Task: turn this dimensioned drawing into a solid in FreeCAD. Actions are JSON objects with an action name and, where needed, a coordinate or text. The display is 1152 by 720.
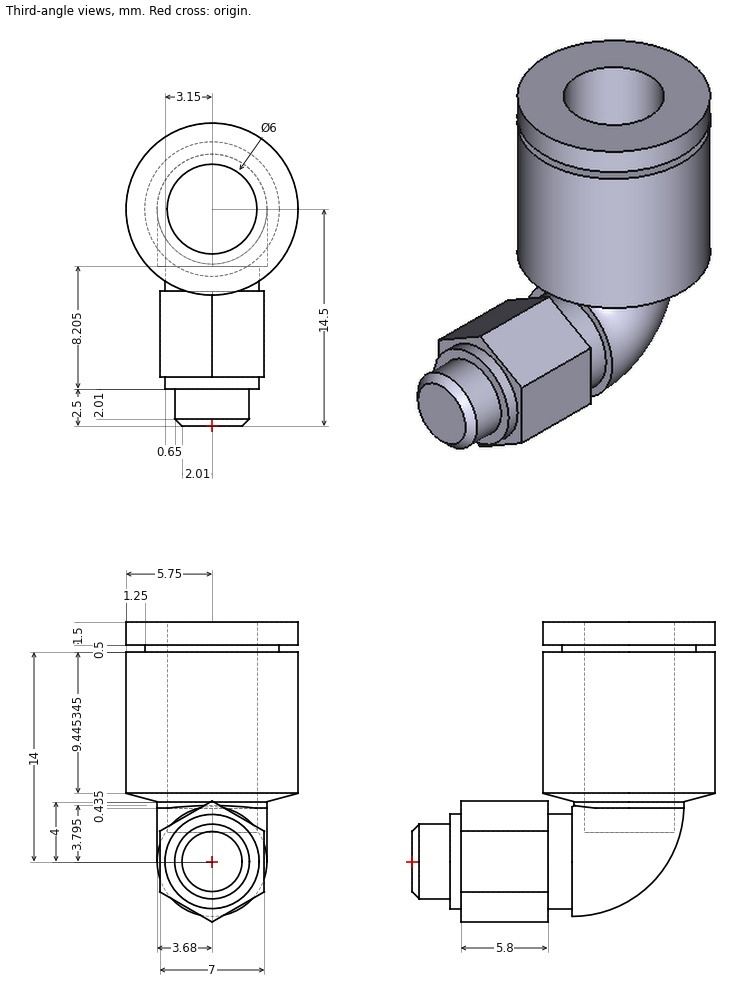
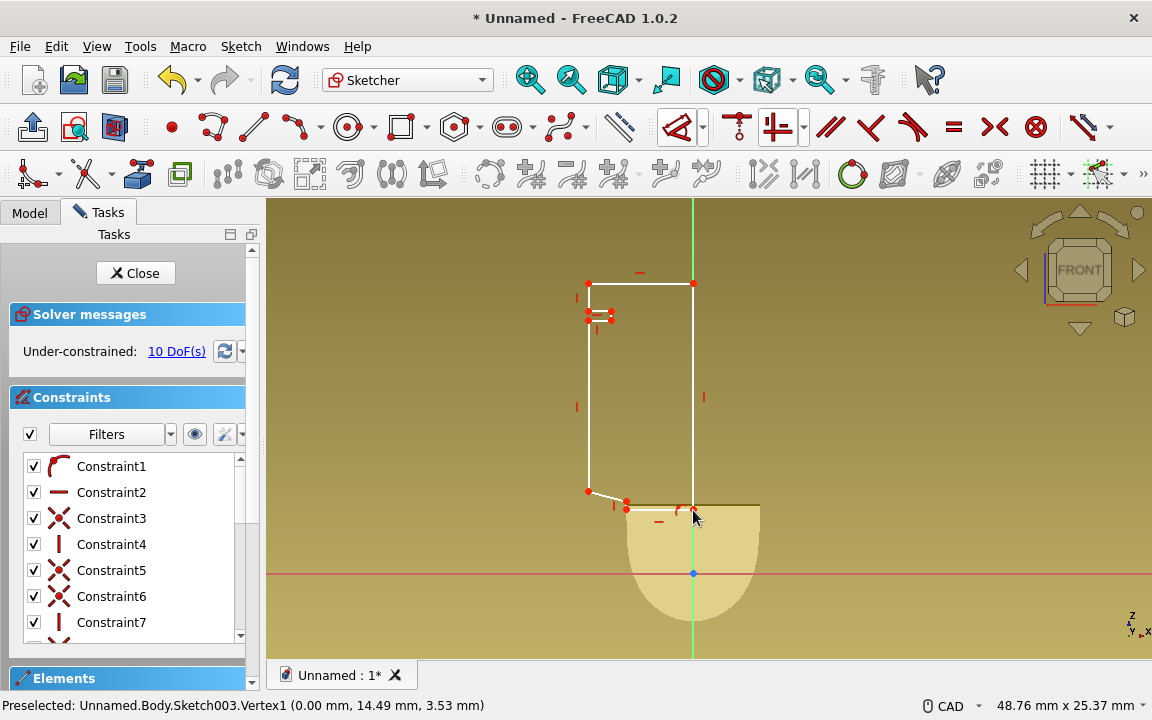
{"action": "scroll", "coordinate": [626, 502], "scroll_direction": "up", "scroll_amount": 3}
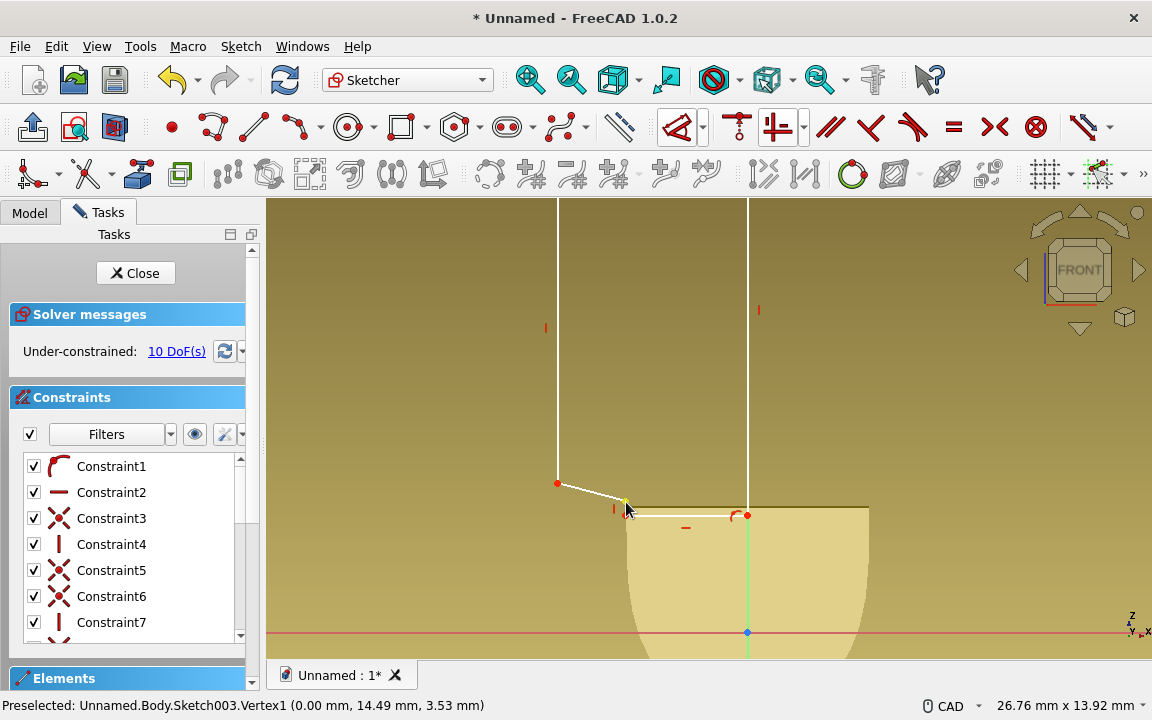
{"action": "left_click", "coordinate": [626, 501]}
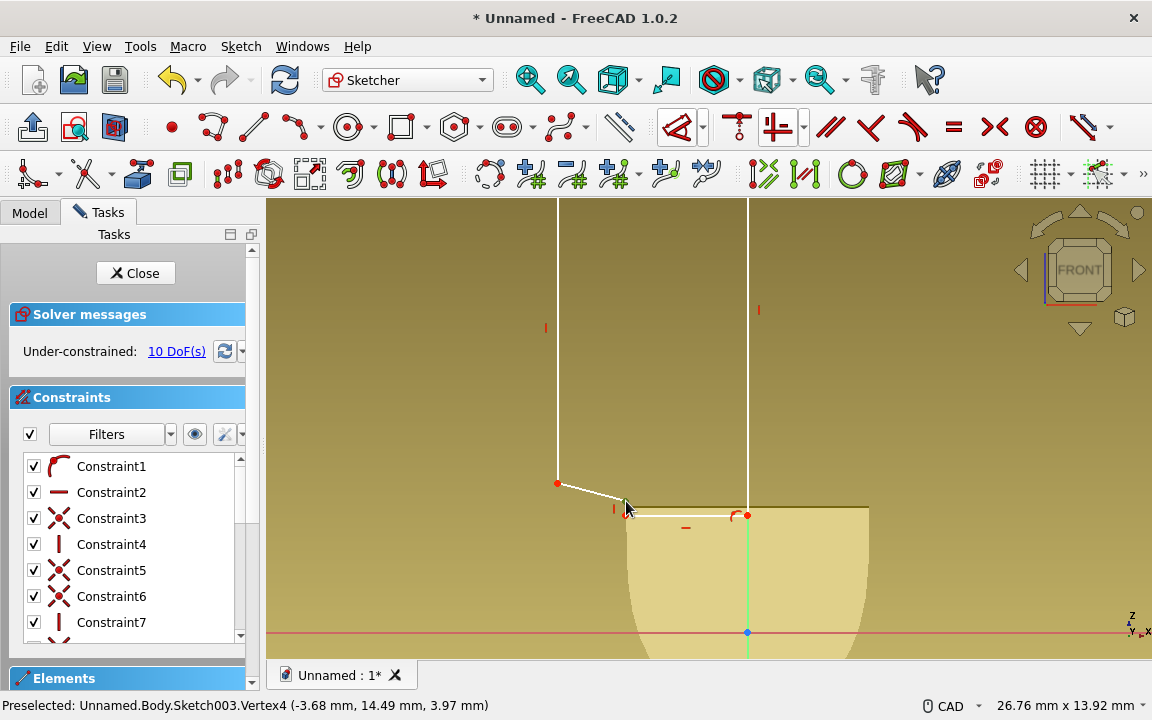
{"action": "key", "text": "i"}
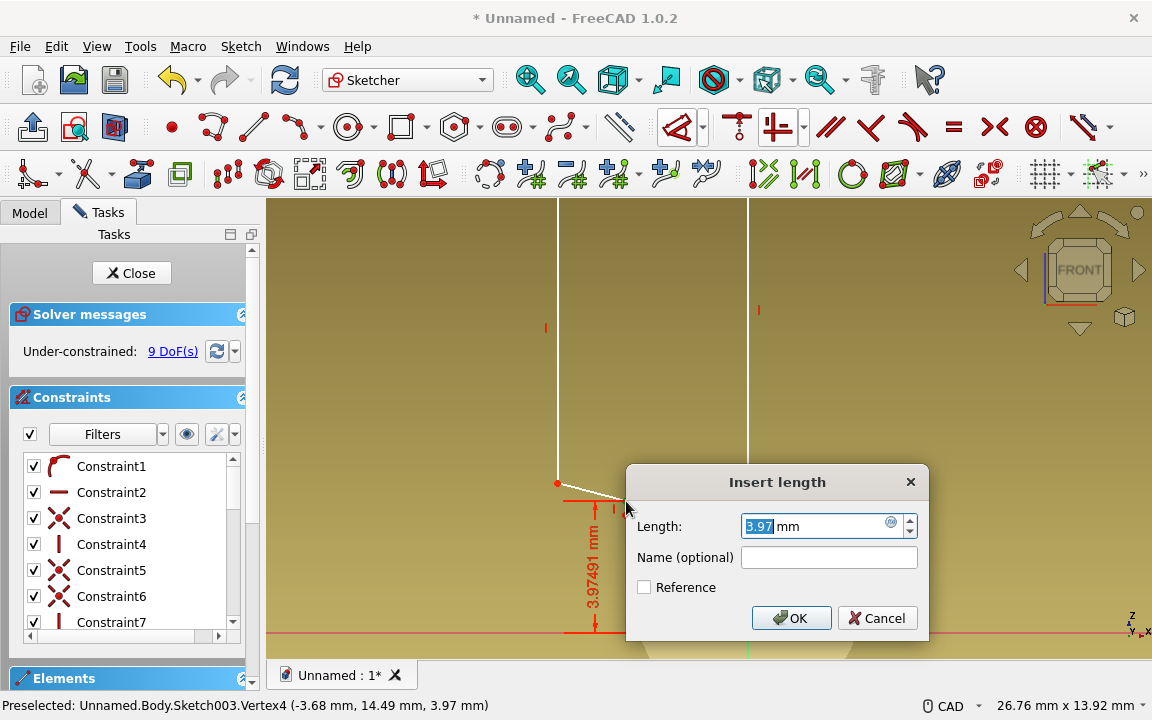
{"action": "type", "text": "4"}
{"action": "key", "text": "Return"}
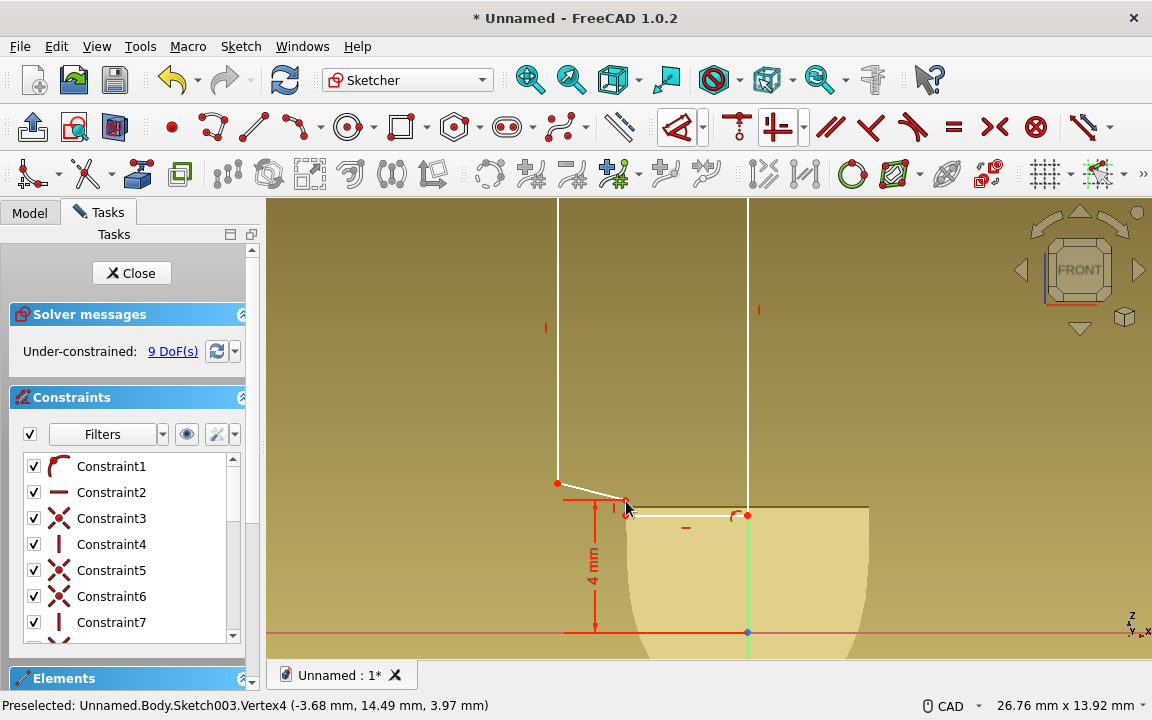
{"action": "scroll", "coordinate": [626, 502], "scroll_direction": "down", "scroll_amount": 3}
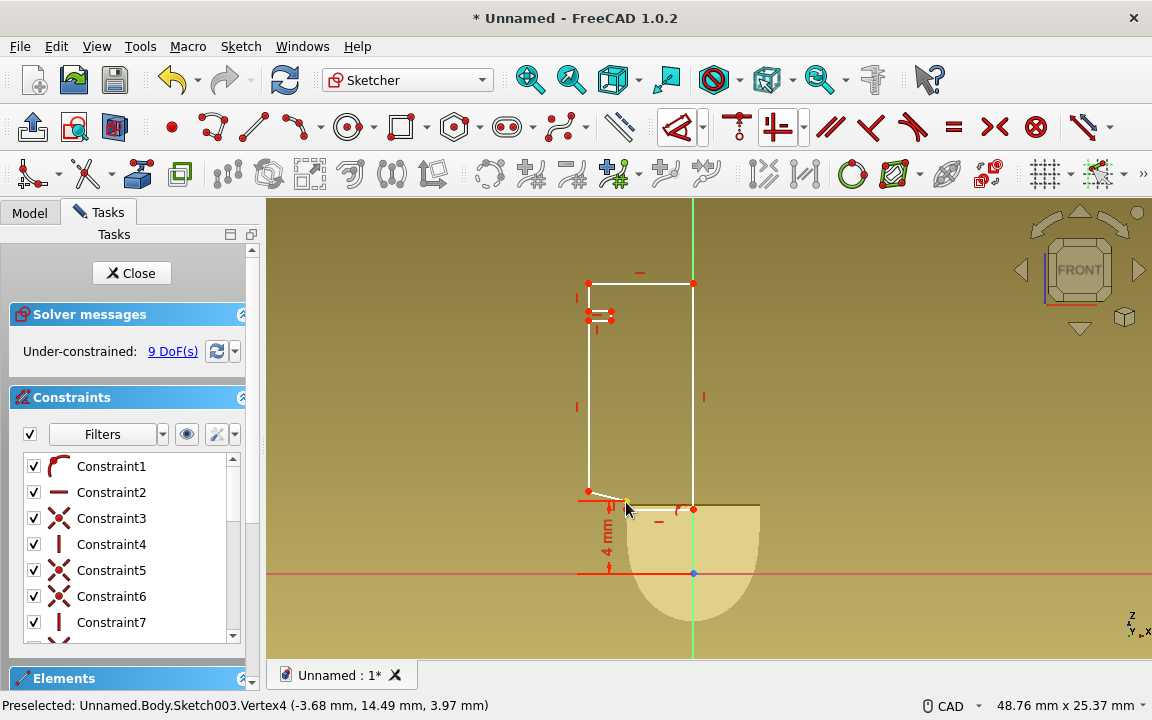
{"action": "scroll", "coordinate": [611, 316], "scroll_direction": "up", "scroll_amount": 8}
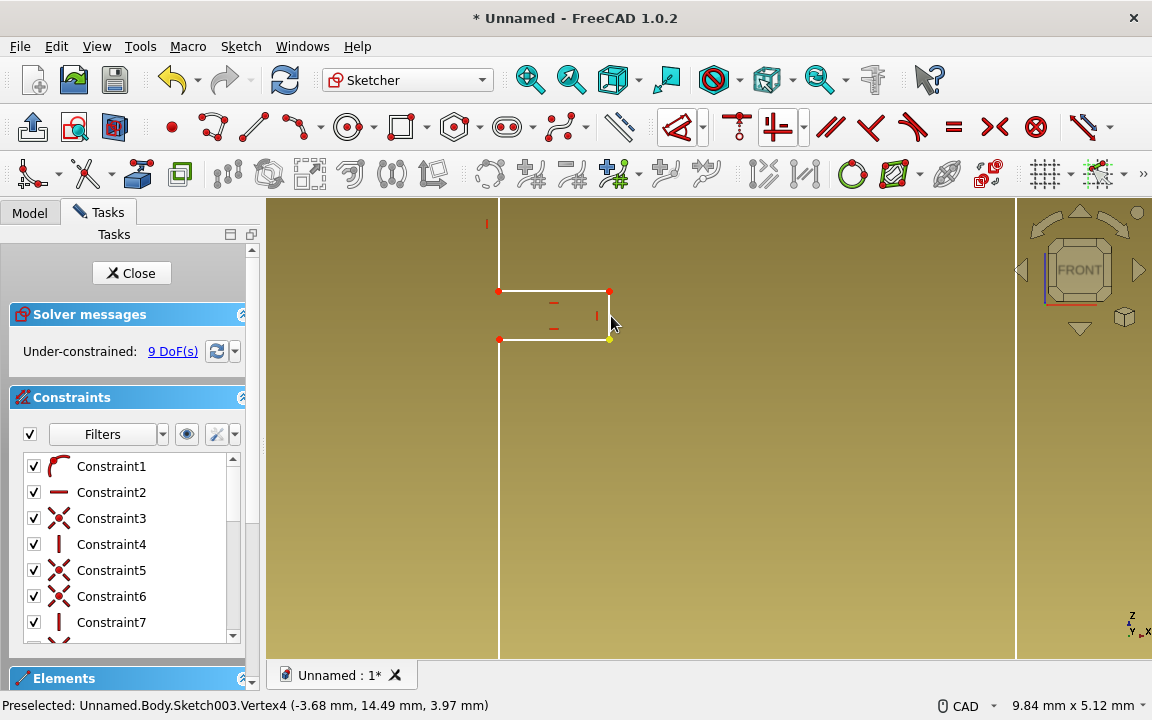
{"action": "left_click", "coordinate": [609, 315]}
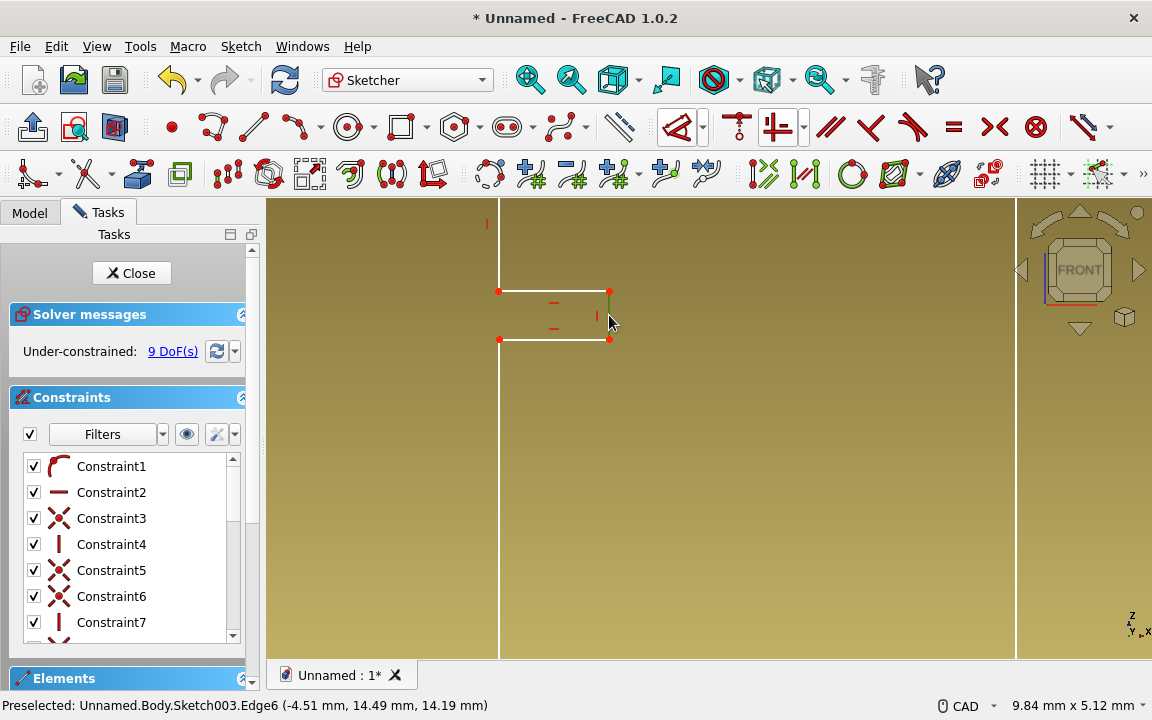
{"action": "left_click", "coordinate": [702, 128]}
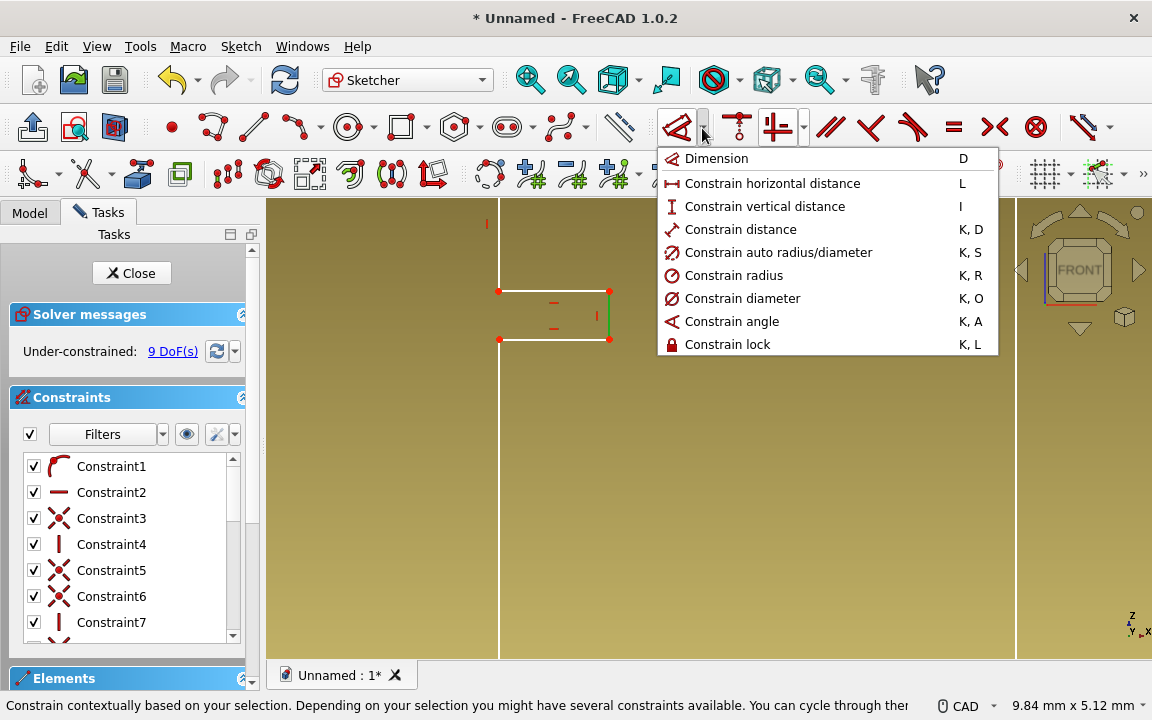
{"action": "left_click", "coordinate": [828, 206]}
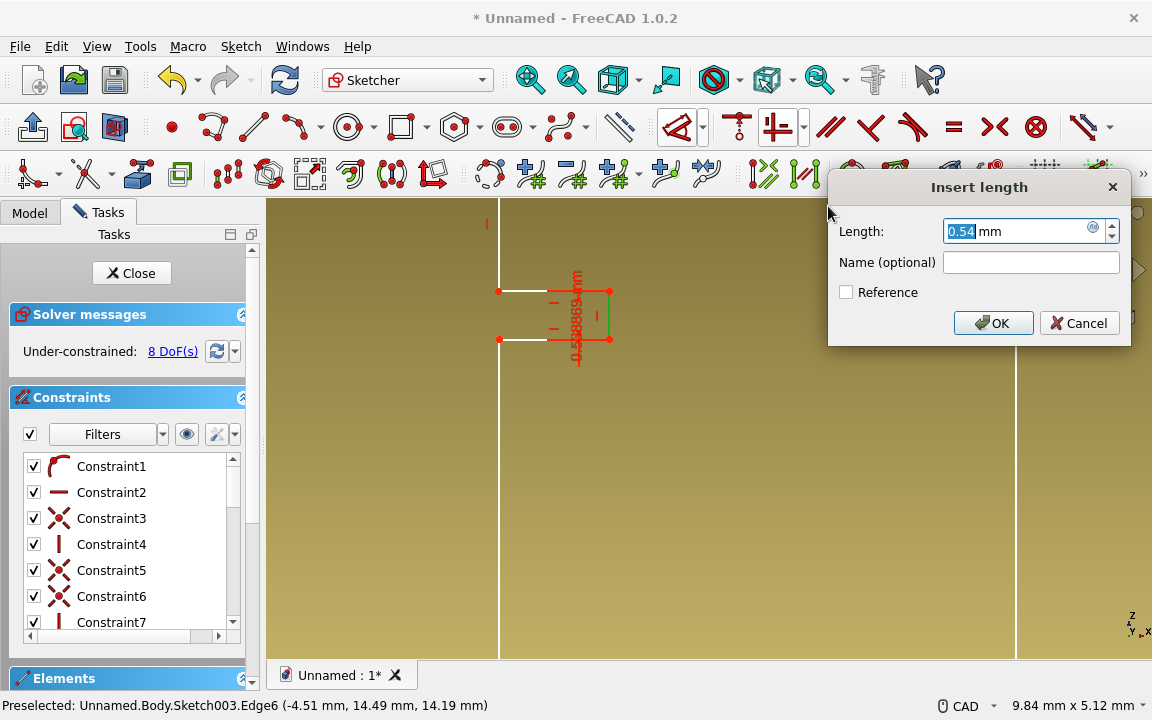
{"action": "type", "text": "0.5"}
{"action": "key", "text": "Return"}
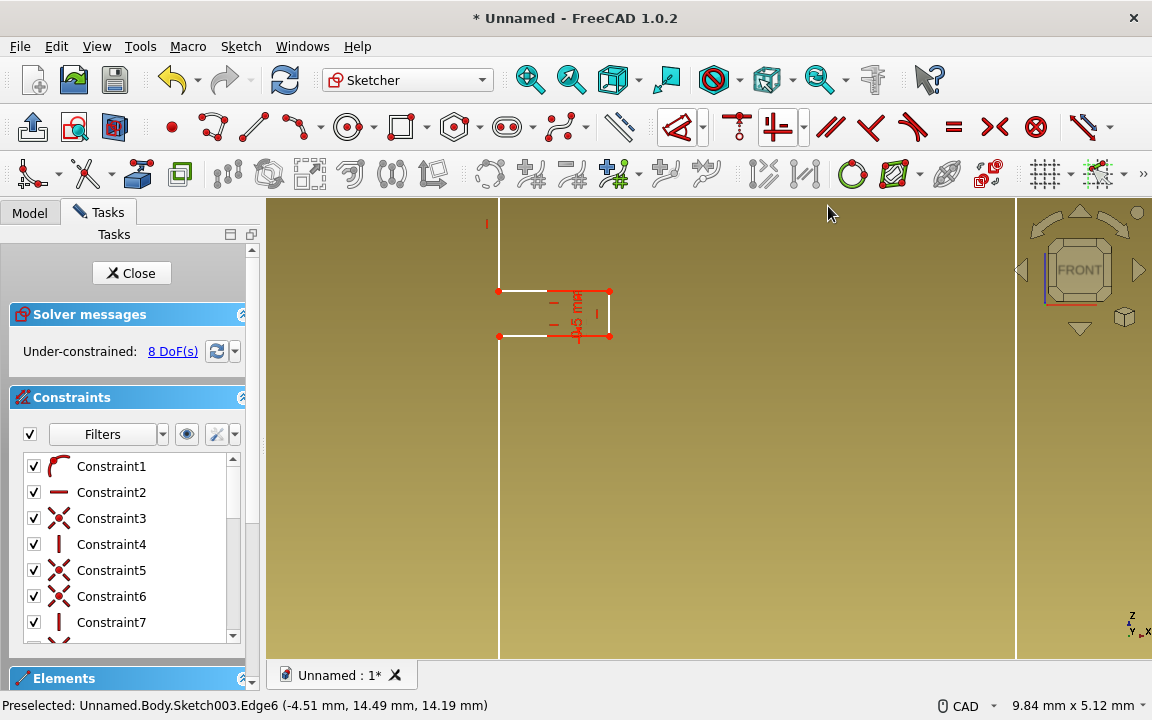
{"action": "scroll", "coordinate": [611, 316], "scroll_direction": "down", "scroll_amount": 8}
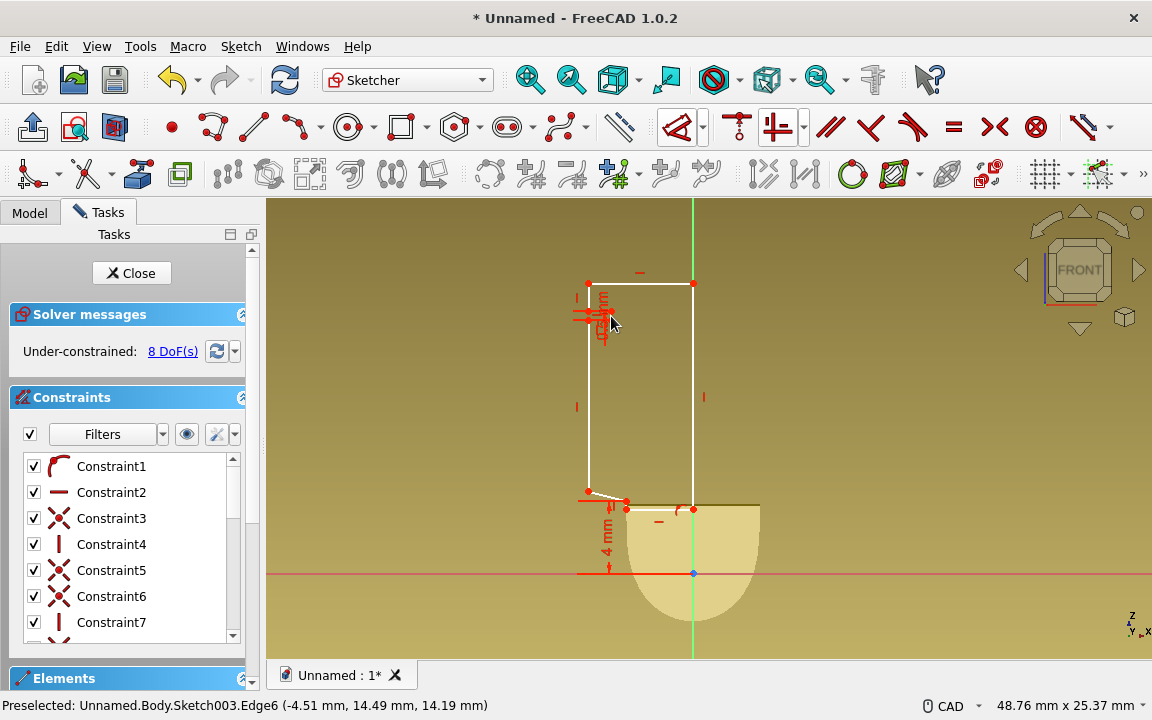
{"action": "scroll", "coordinate": [589, 303], "scroll_direction": "up", "scroll_amount": 3}